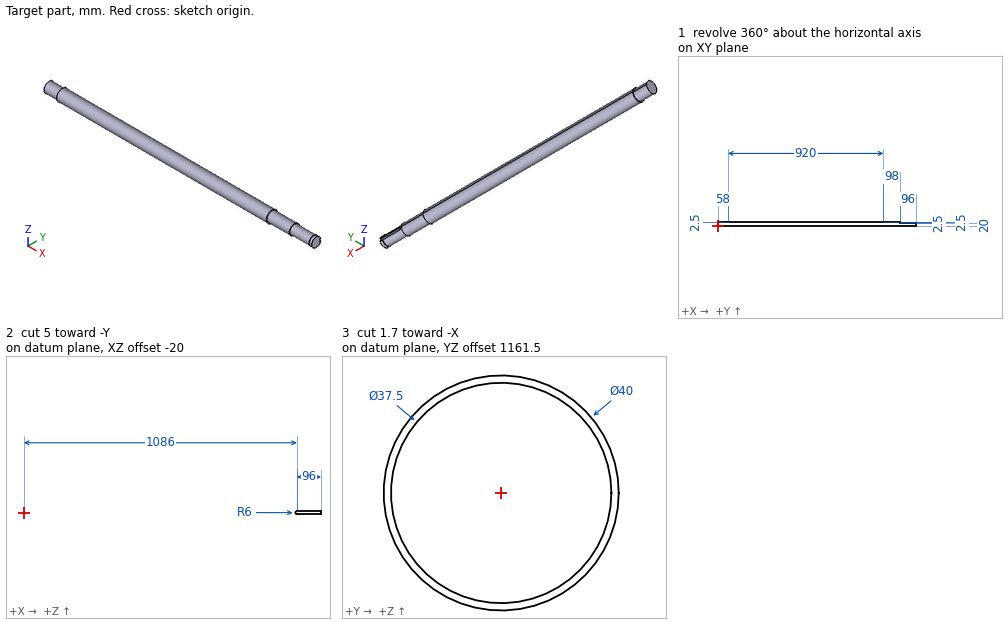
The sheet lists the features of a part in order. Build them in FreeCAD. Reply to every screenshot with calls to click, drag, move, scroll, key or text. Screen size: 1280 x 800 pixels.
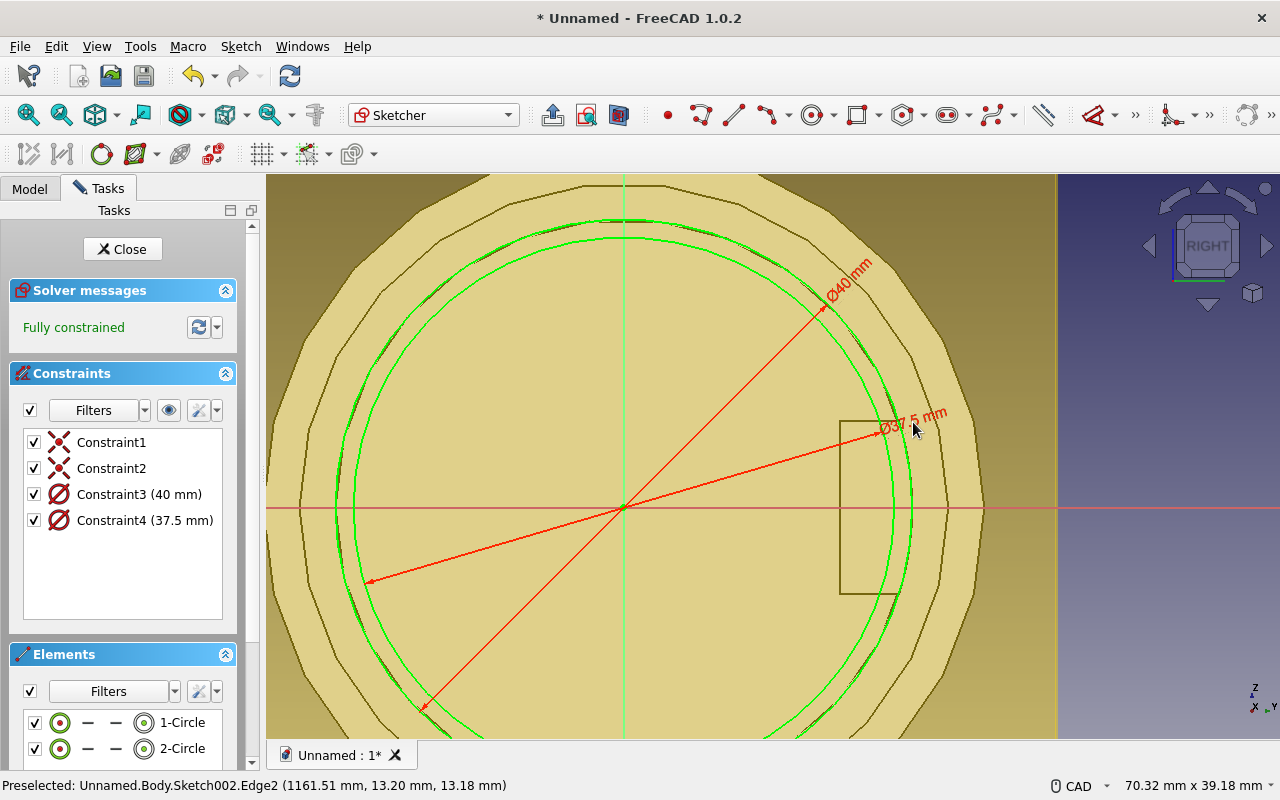
click(123, 249)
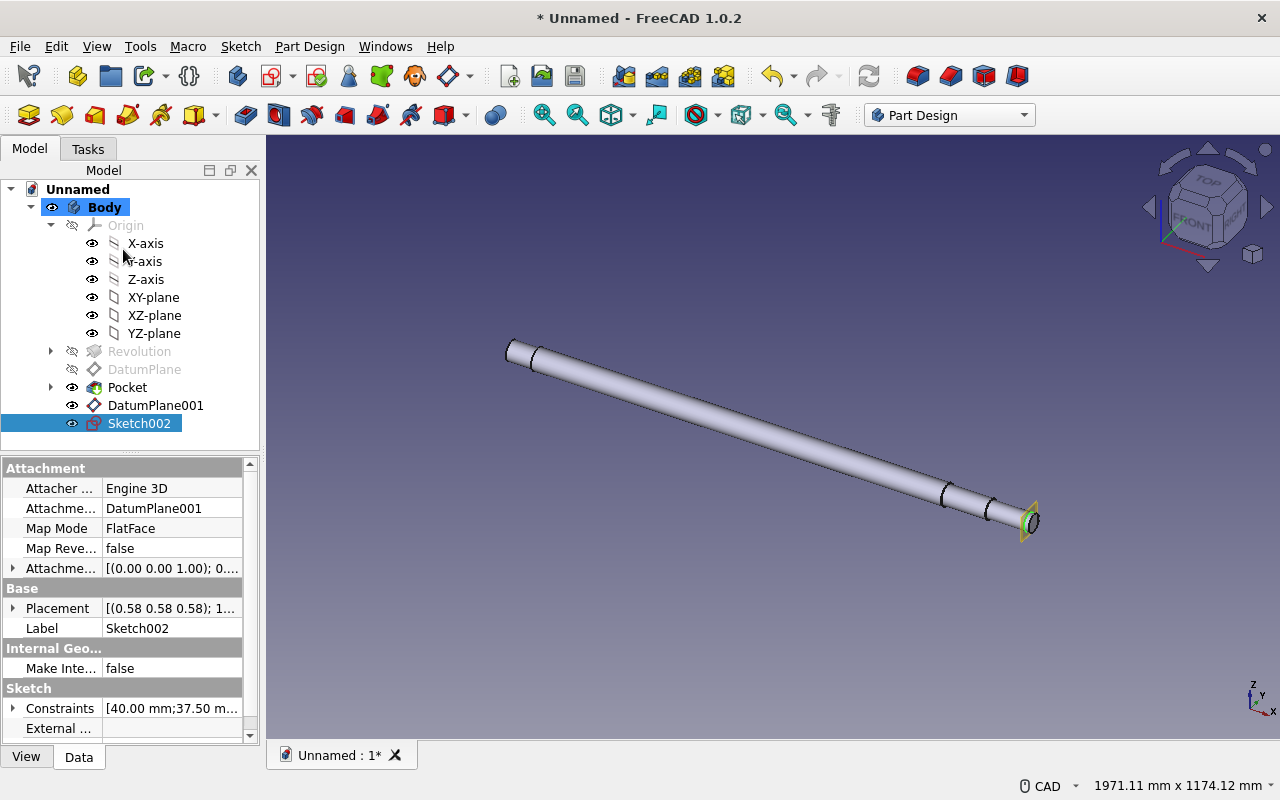
click(246, 116)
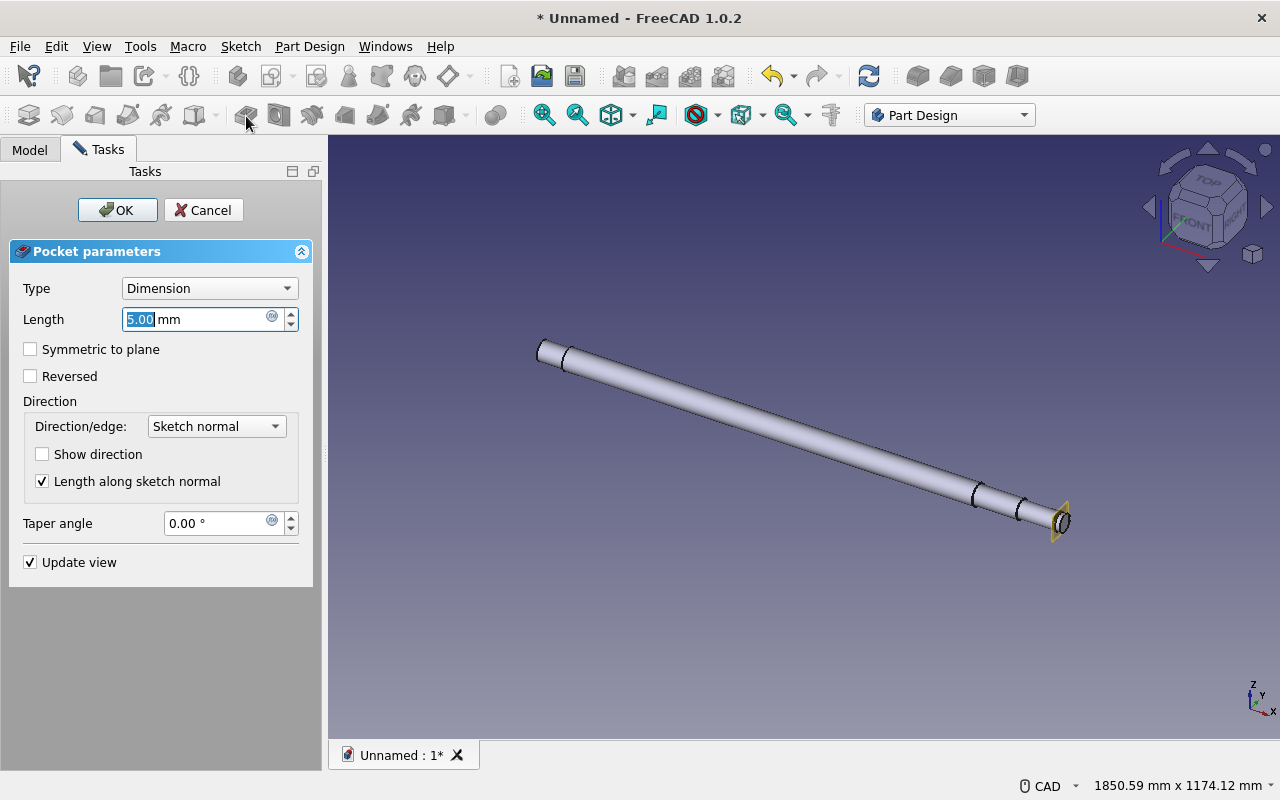
text(1.7)
key(Tab)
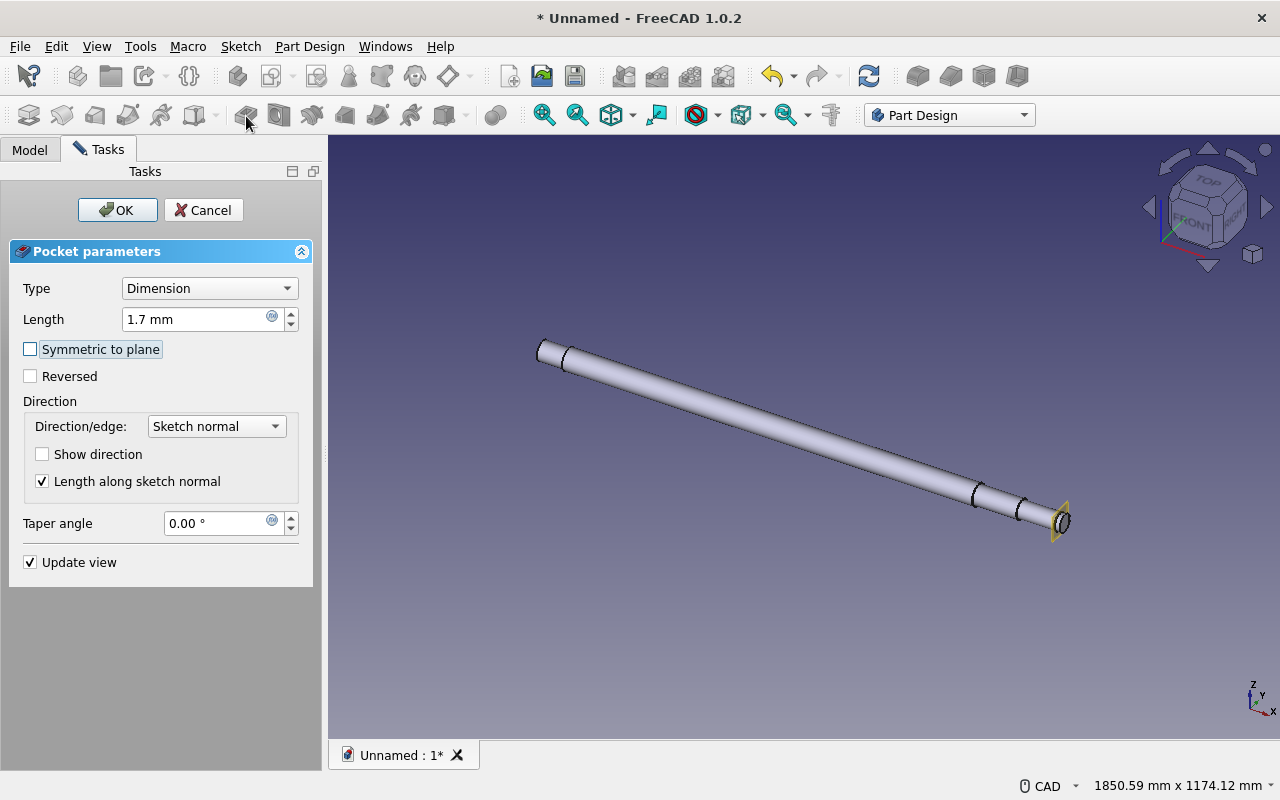
click(118, 210)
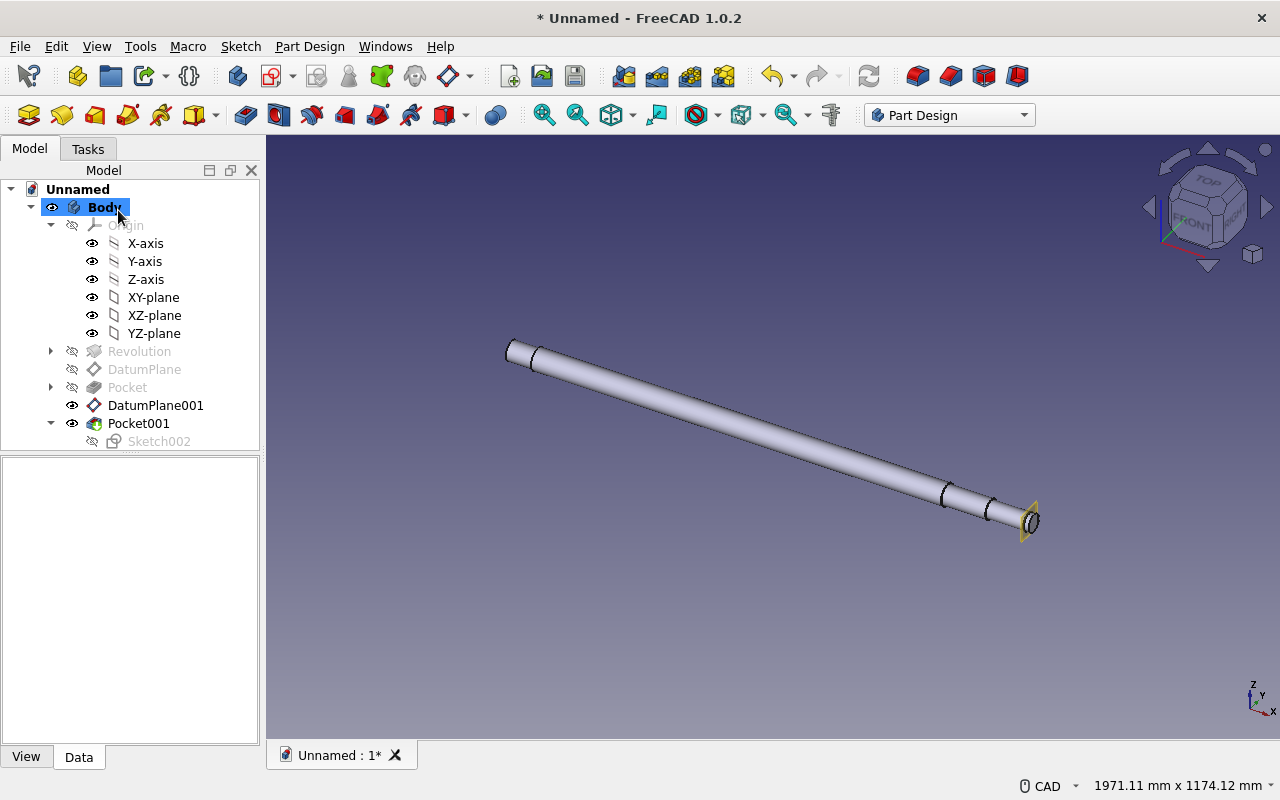
click(117, 405)
key(space)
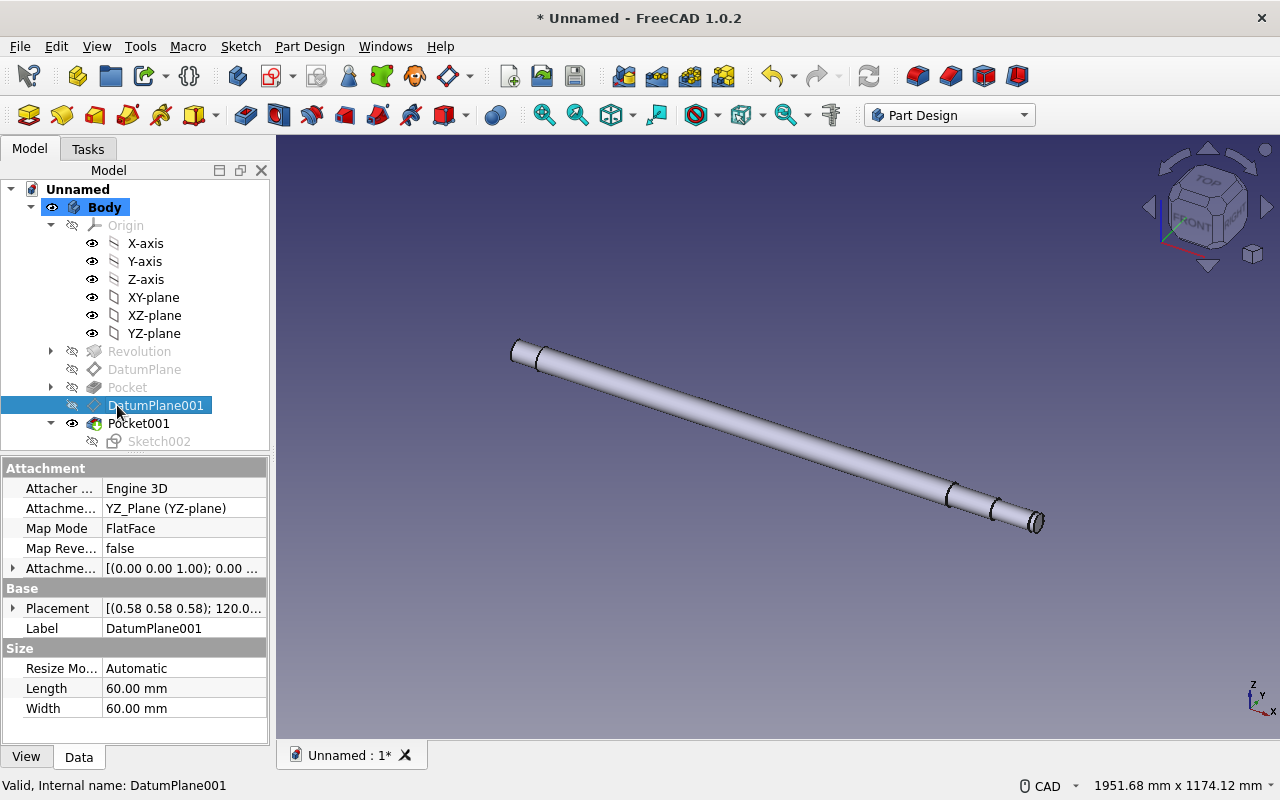
key(0)